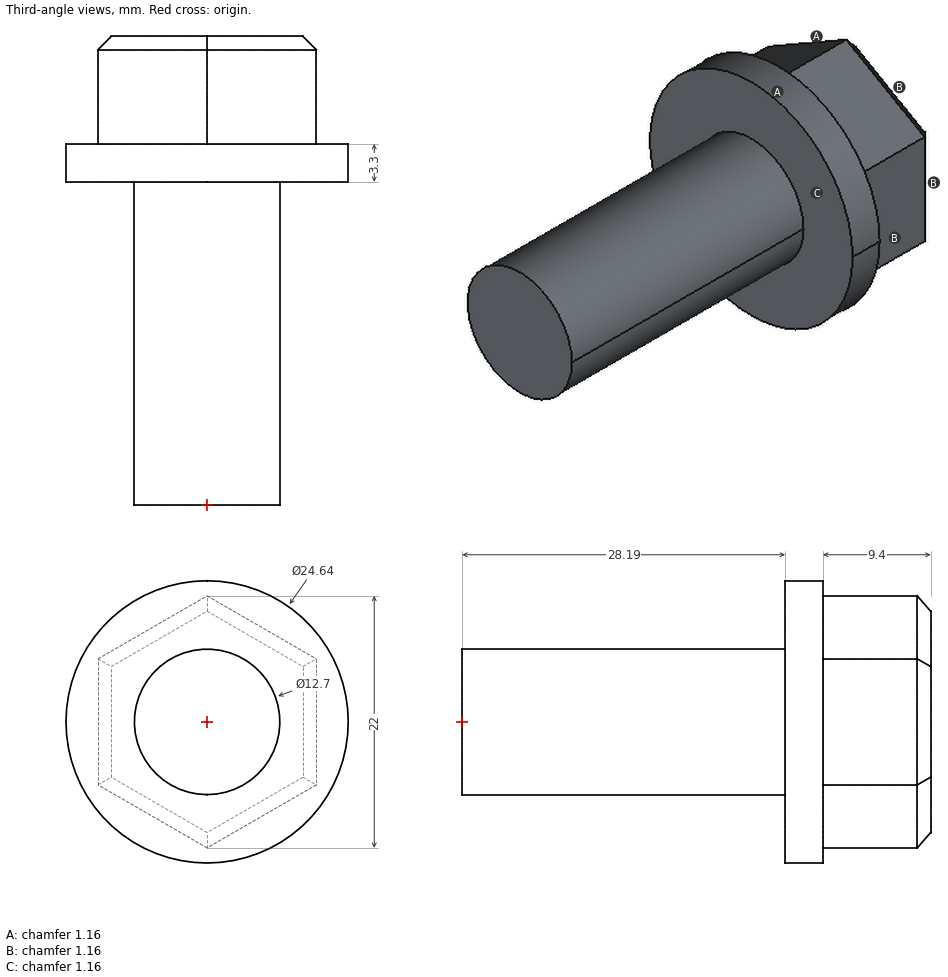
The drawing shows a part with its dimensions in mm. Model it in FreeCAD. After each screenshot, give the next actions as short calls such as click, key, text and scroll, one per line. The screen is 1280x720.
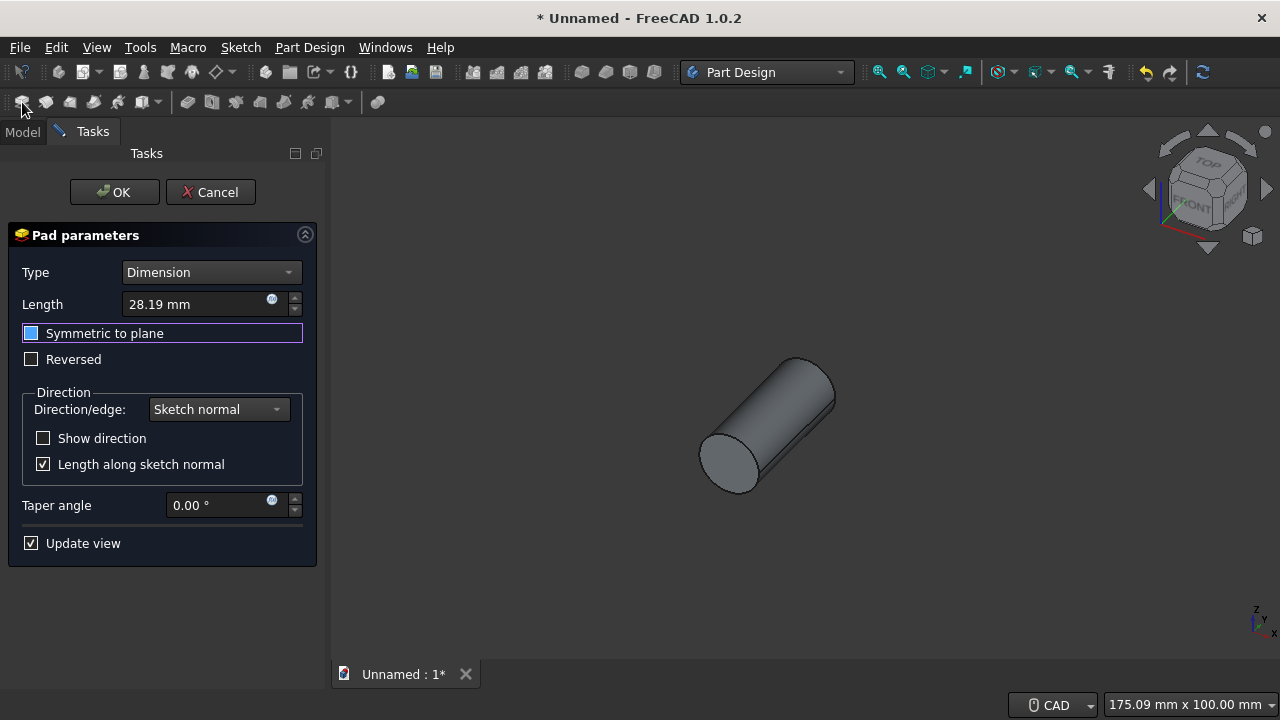
click(30, 359)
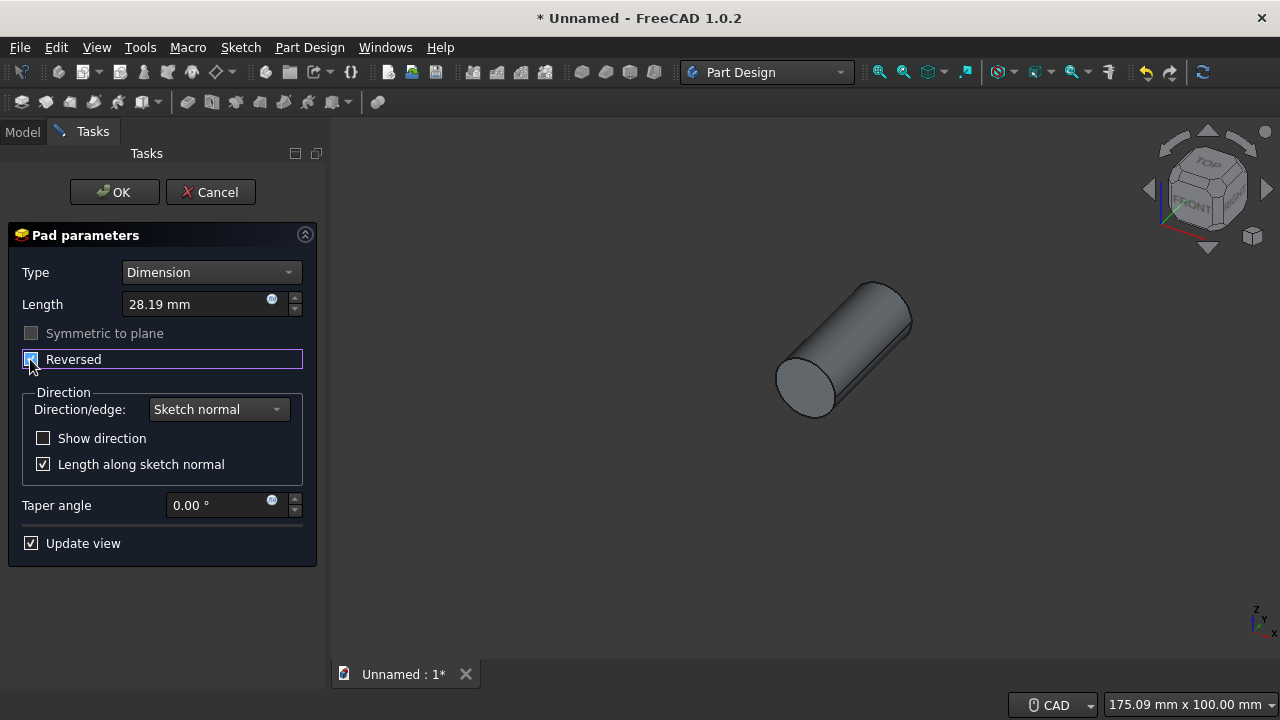
click(115, 192)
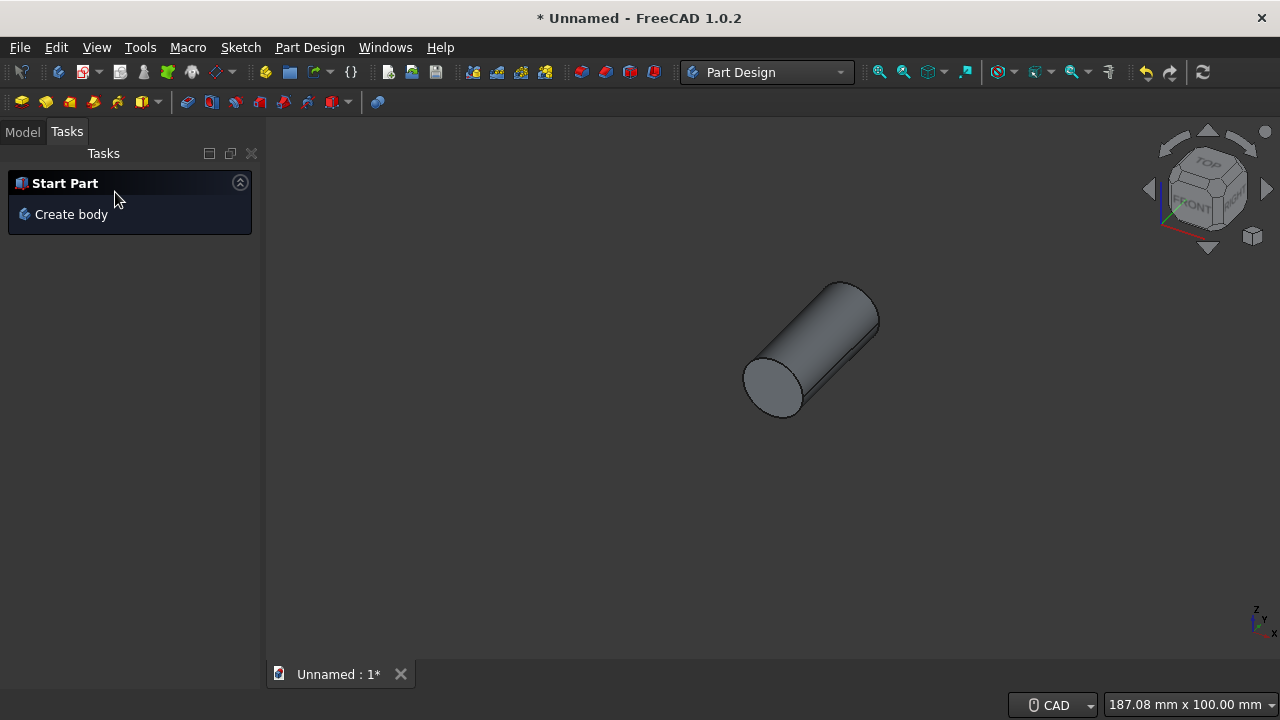
click(880, 72)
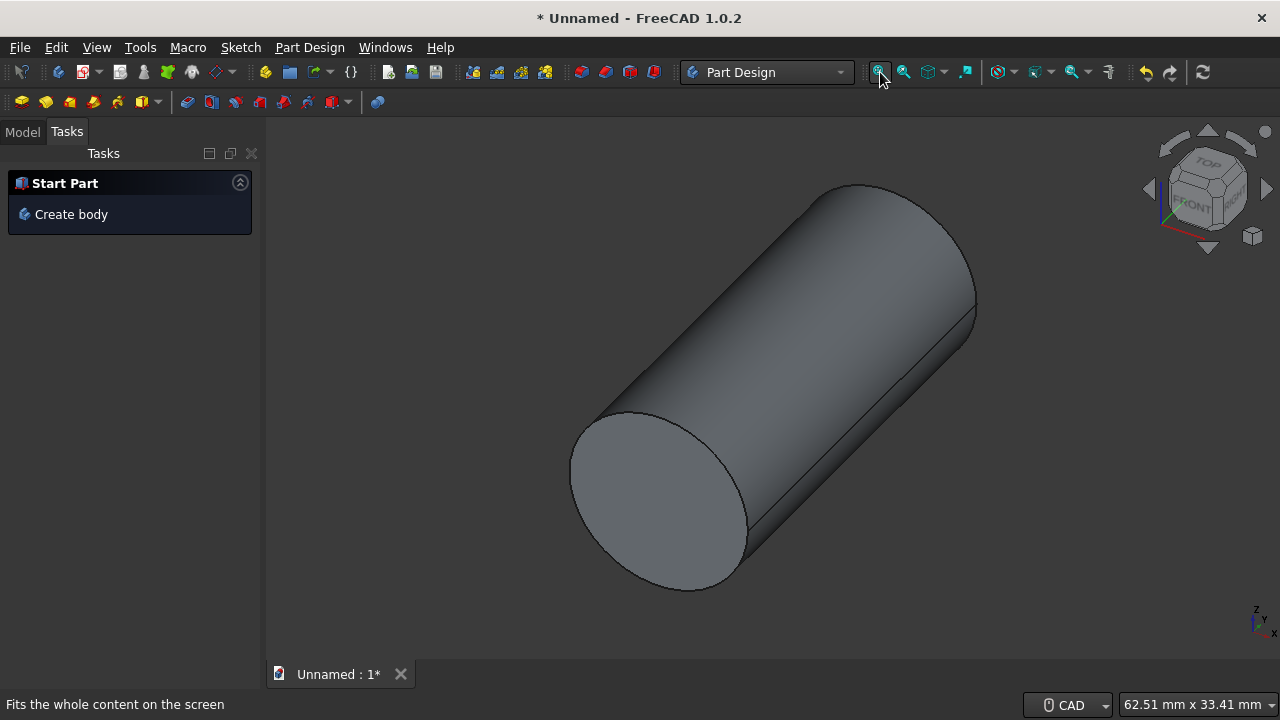
key(4)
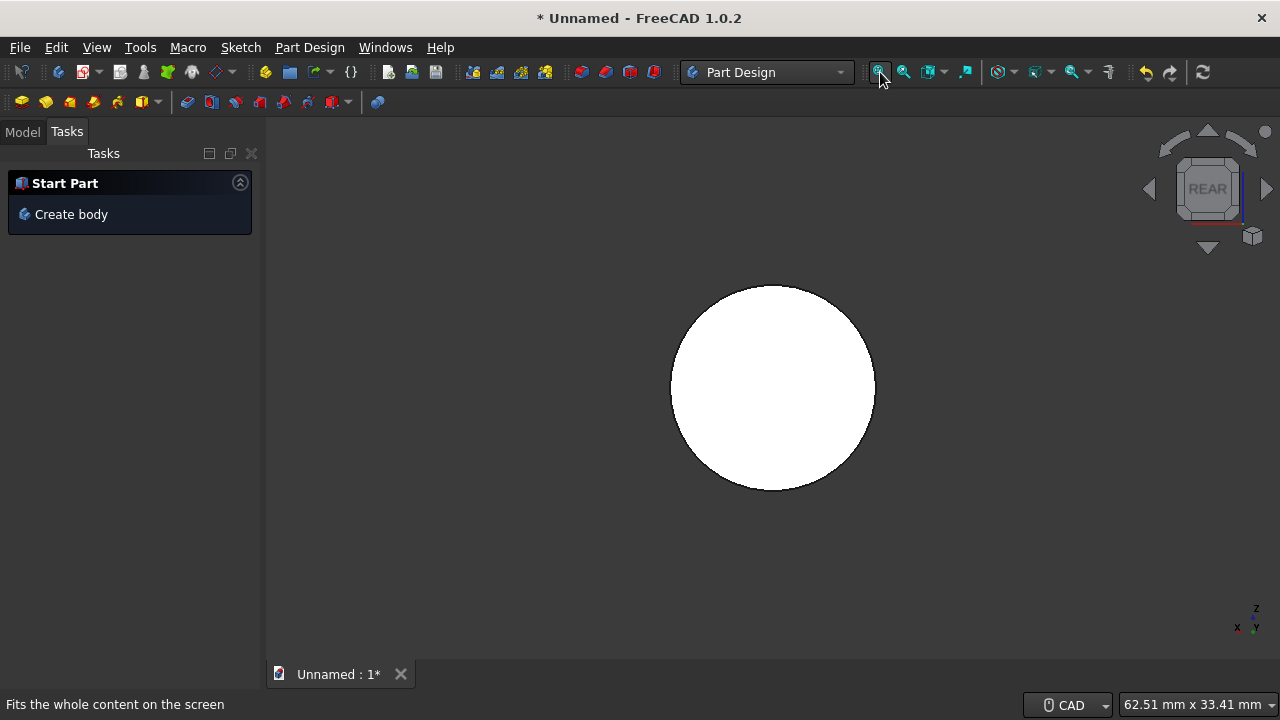
click(880, 72)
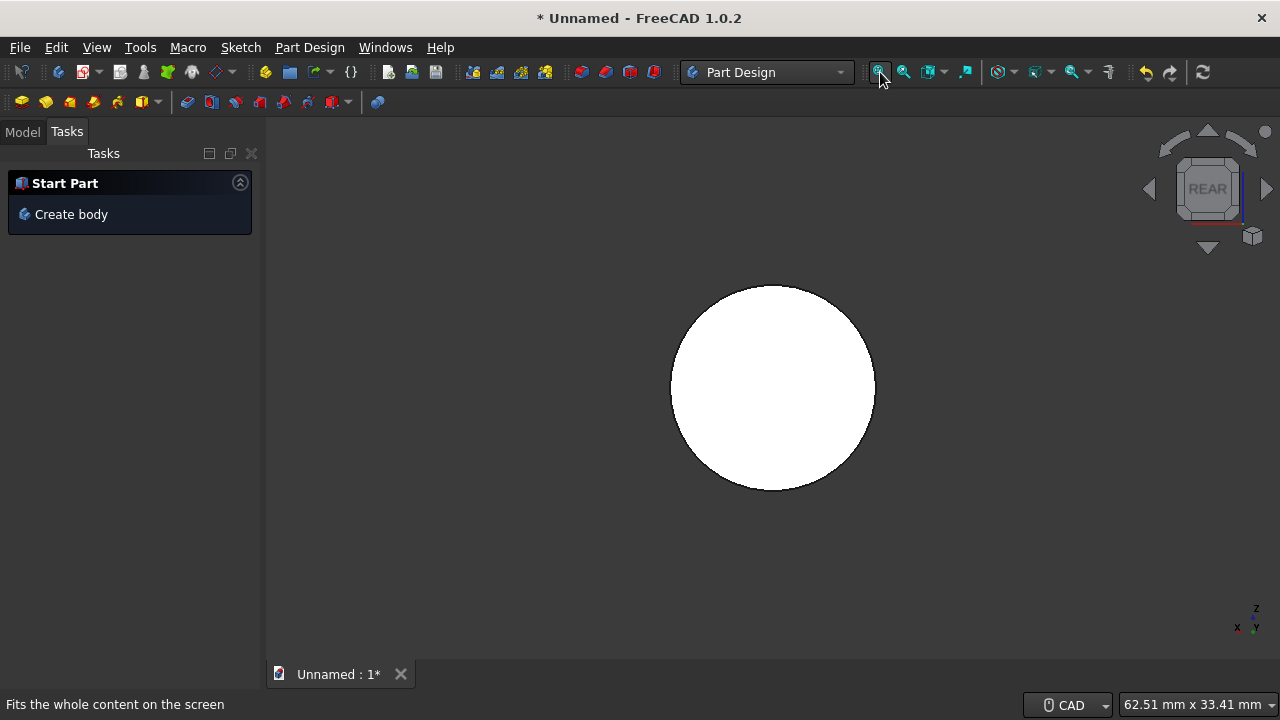
click(773, 387)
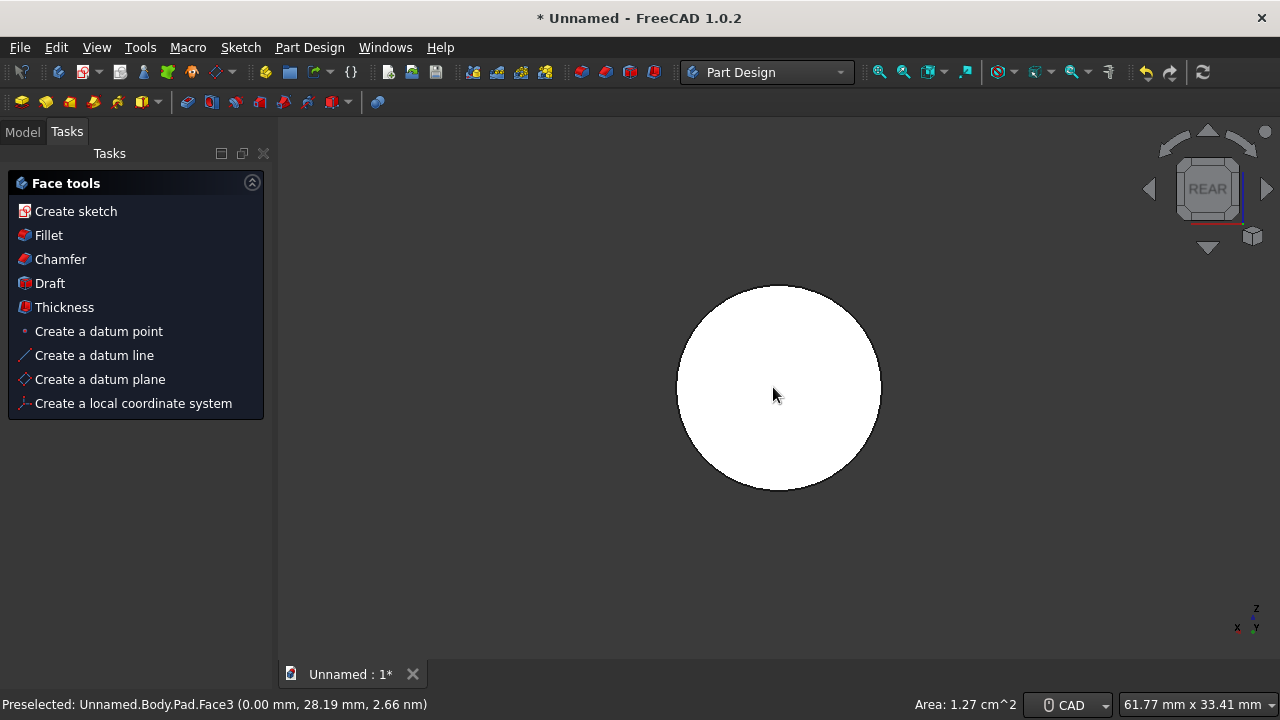
click(84, 72)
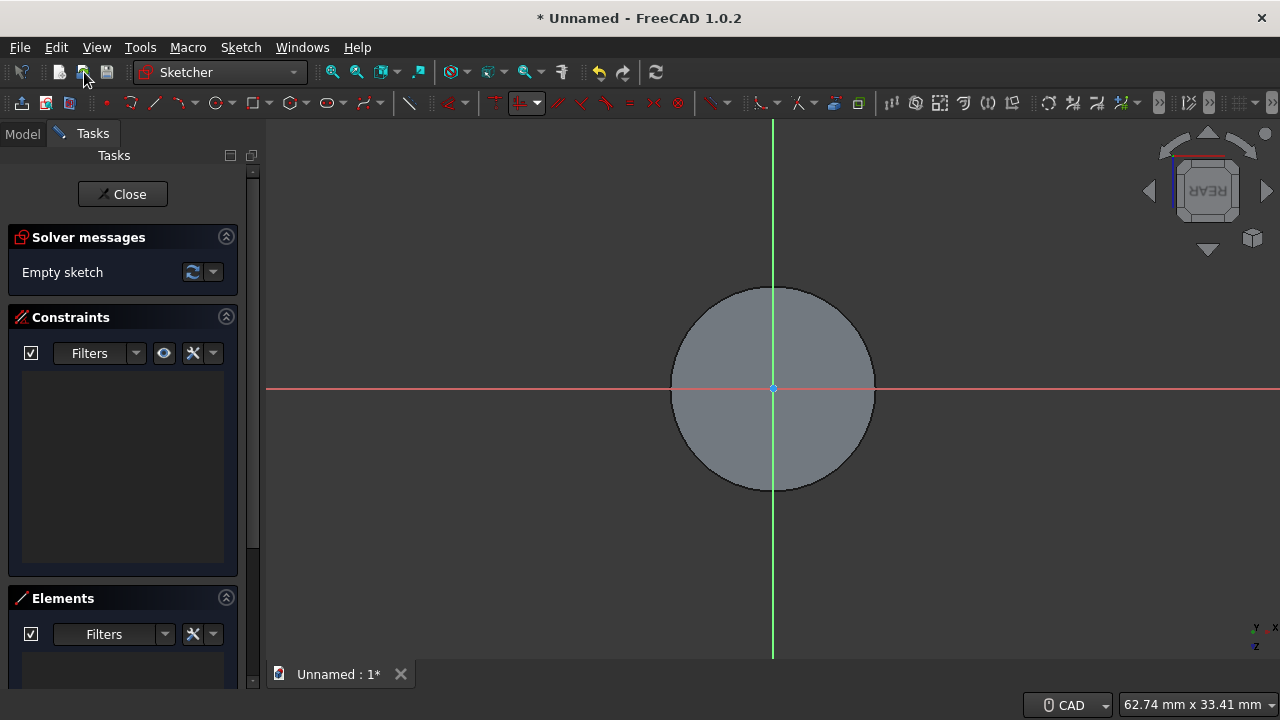
click(216, 104)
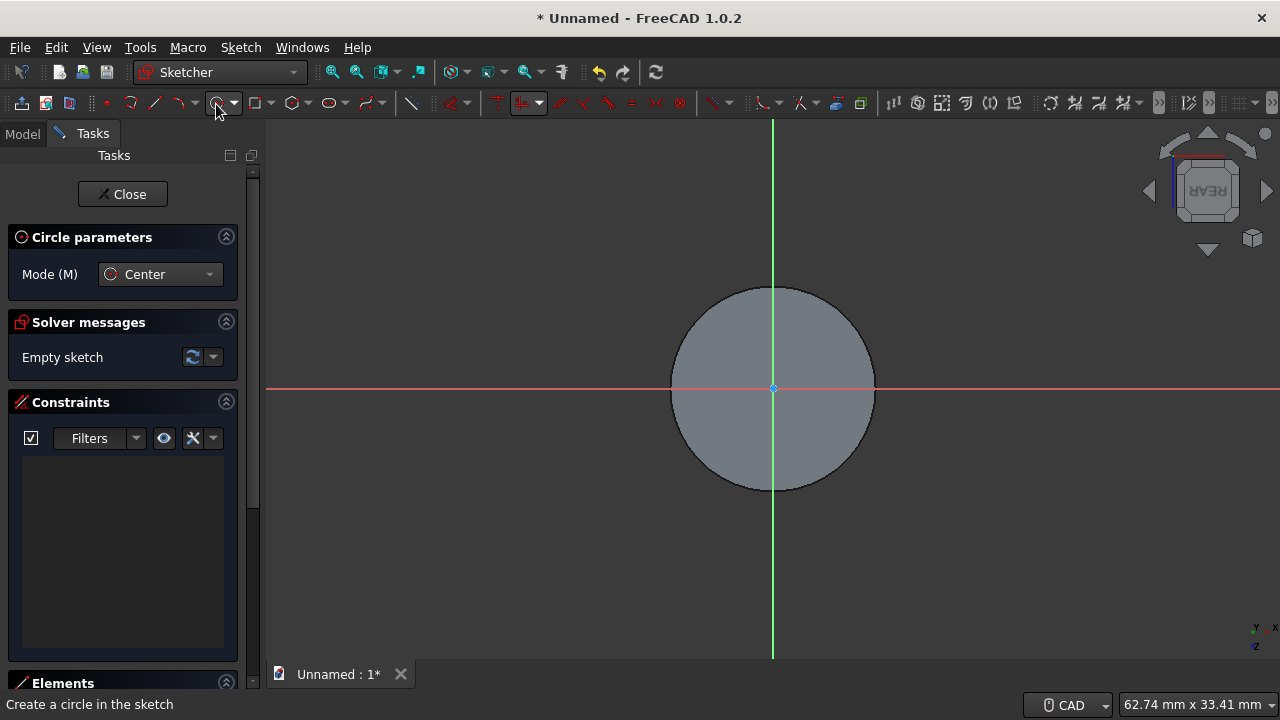
click(773, 389)
move(914, 248)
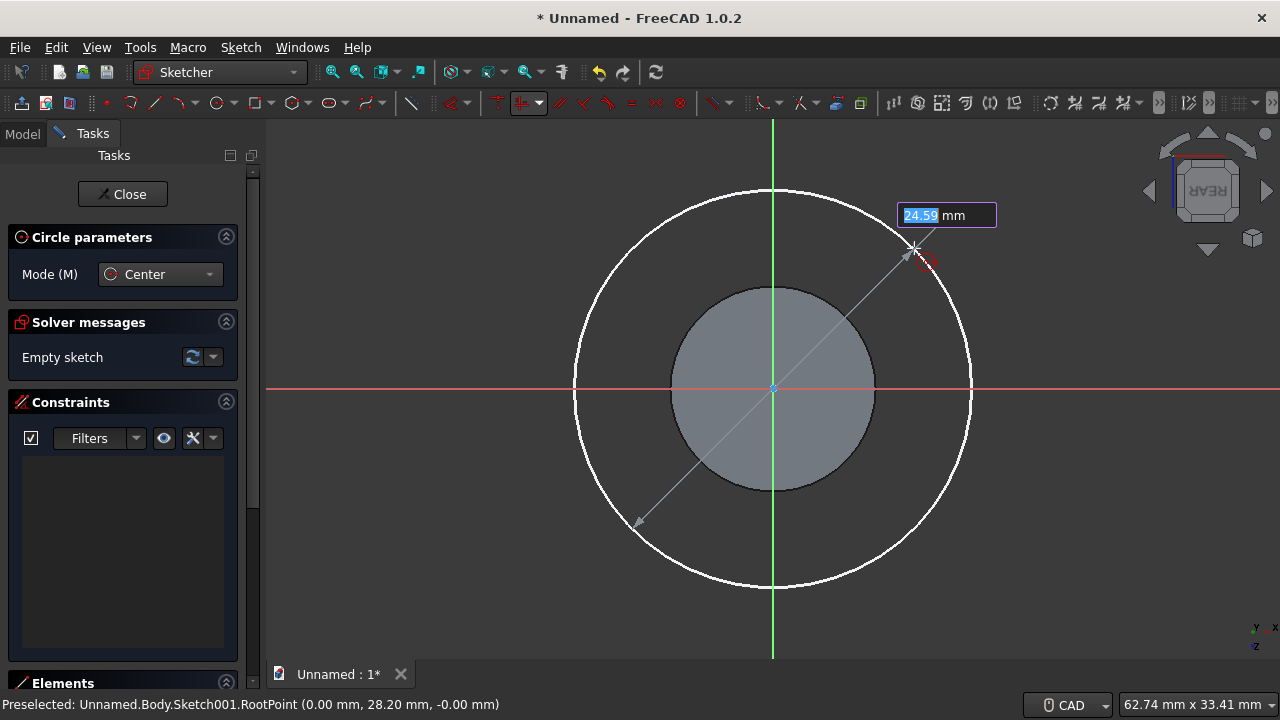
text(24.64)
key(Return)
key(Escape)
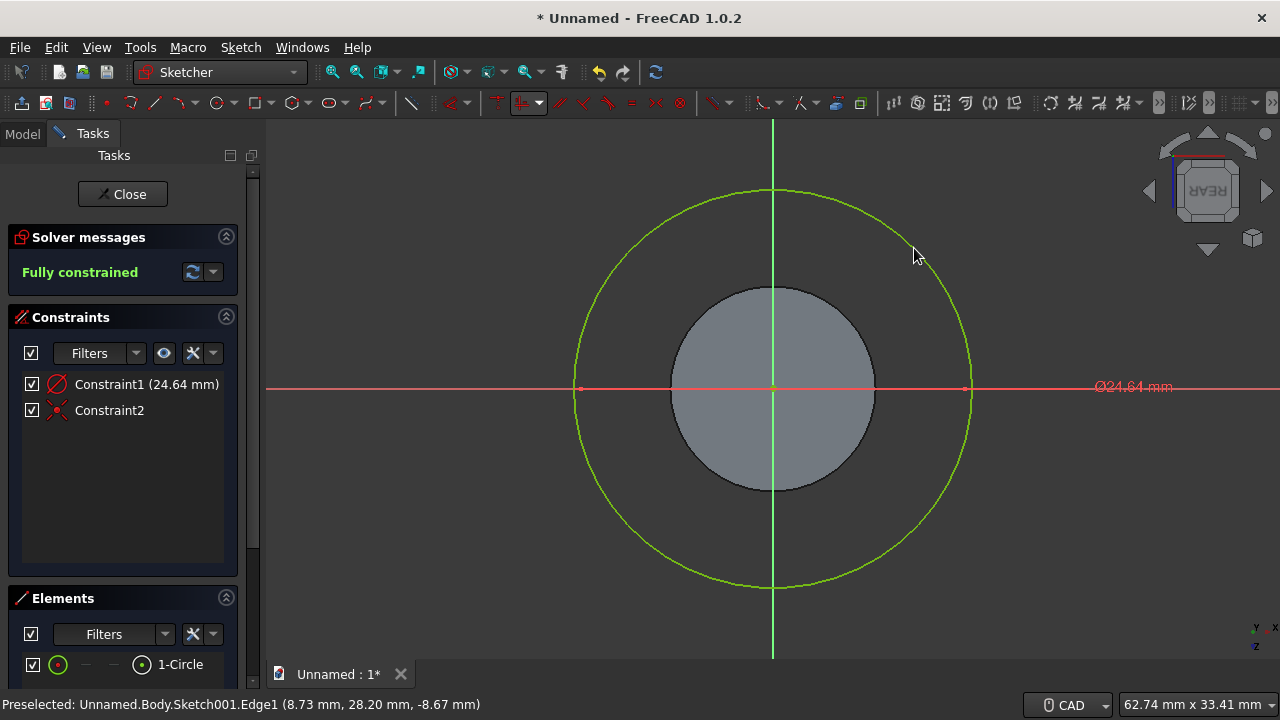
click(123, 194)